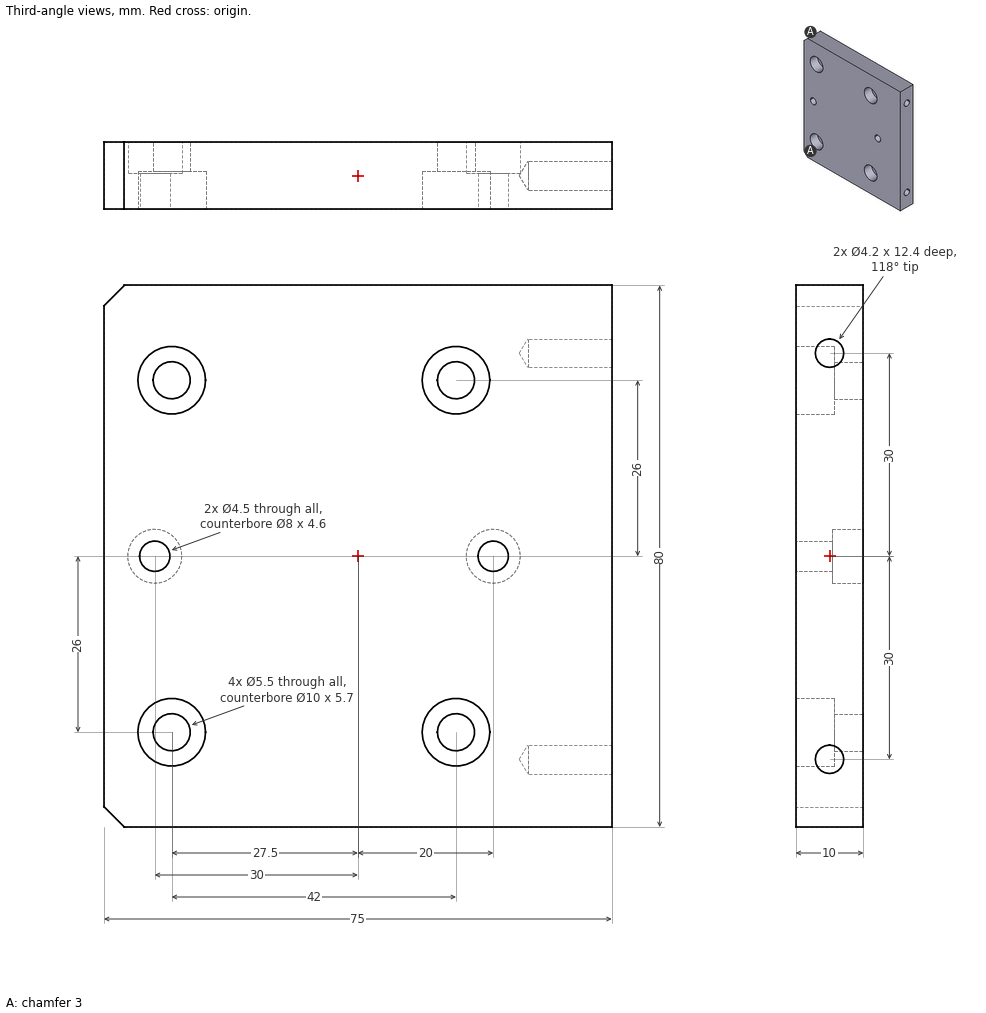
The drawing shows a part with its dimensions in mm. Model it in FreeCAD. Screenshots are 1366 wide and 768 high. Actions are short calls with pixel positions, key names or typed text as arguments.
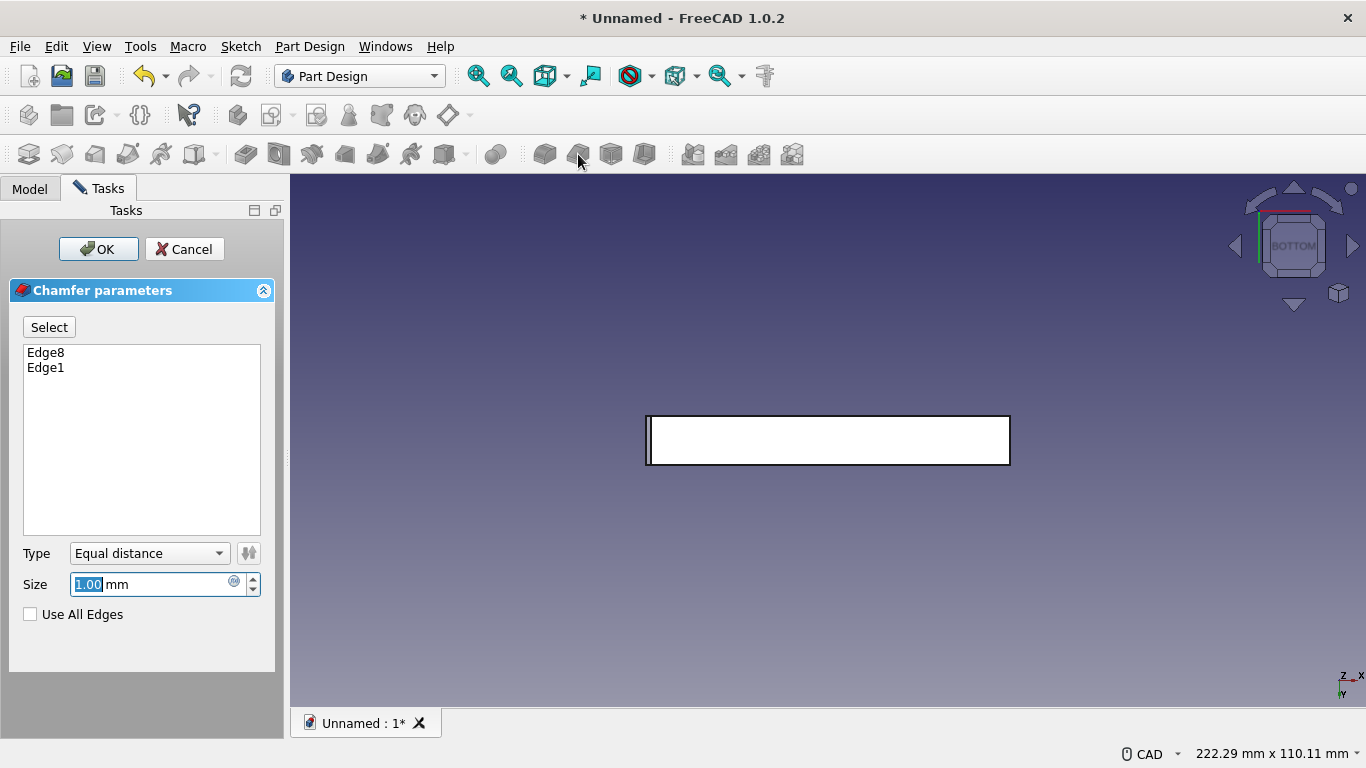
text(3)
key(Tab)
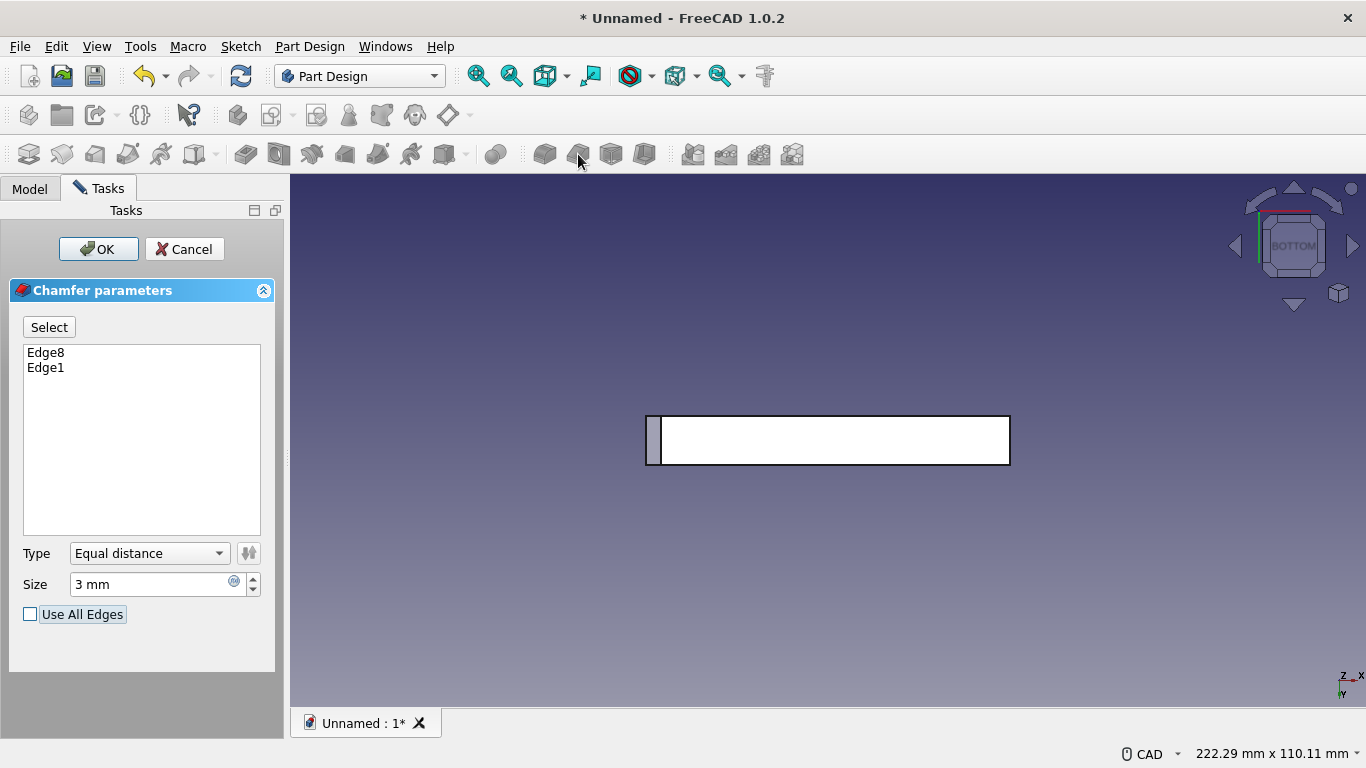
click(99, 249)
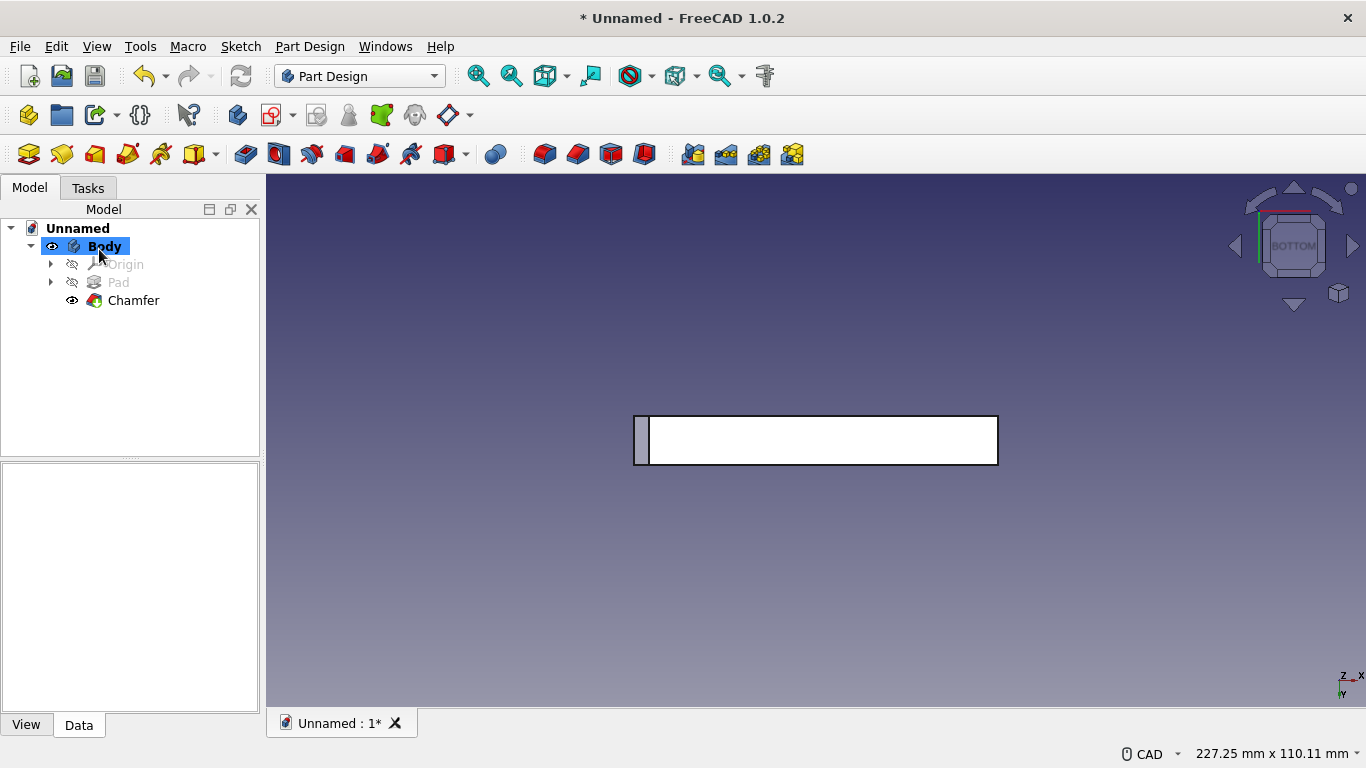
click(479, 76)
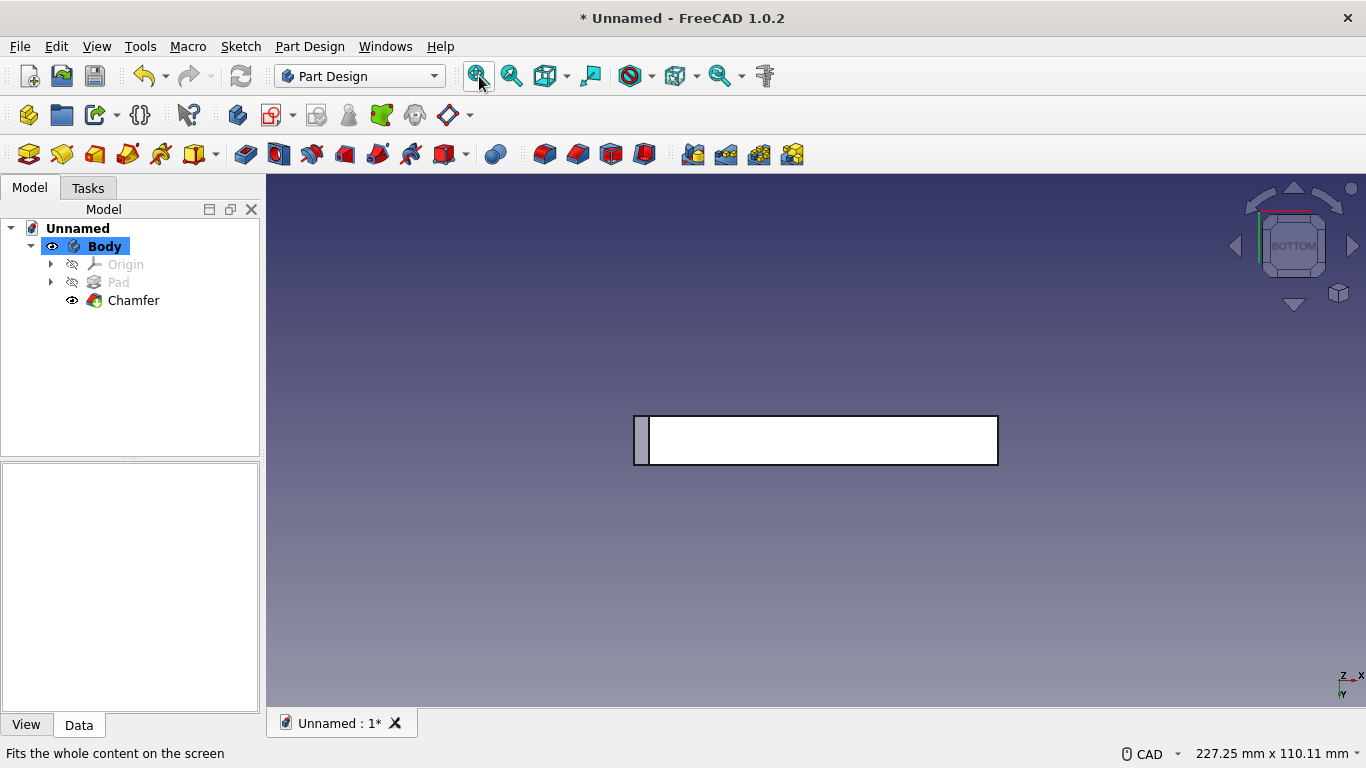
key(0)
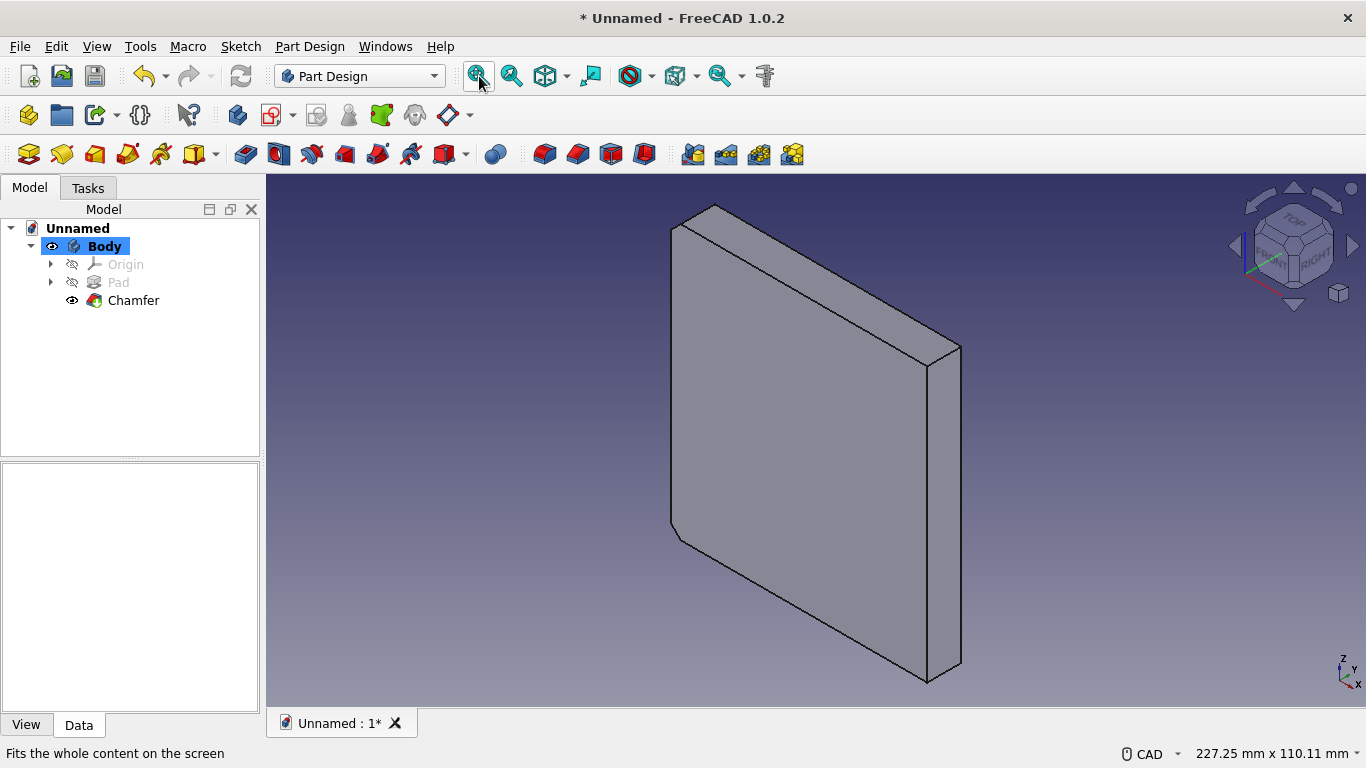
click(944, 468)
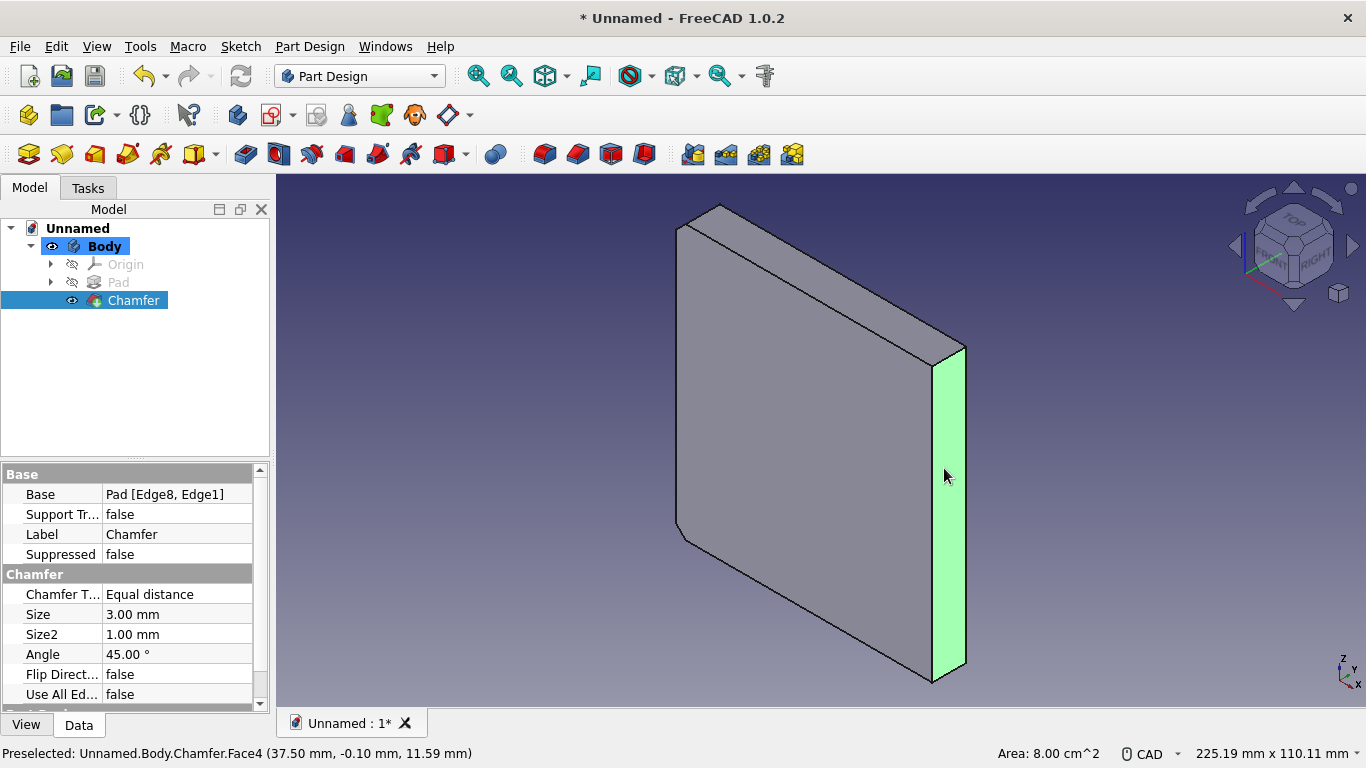
click(270, 116)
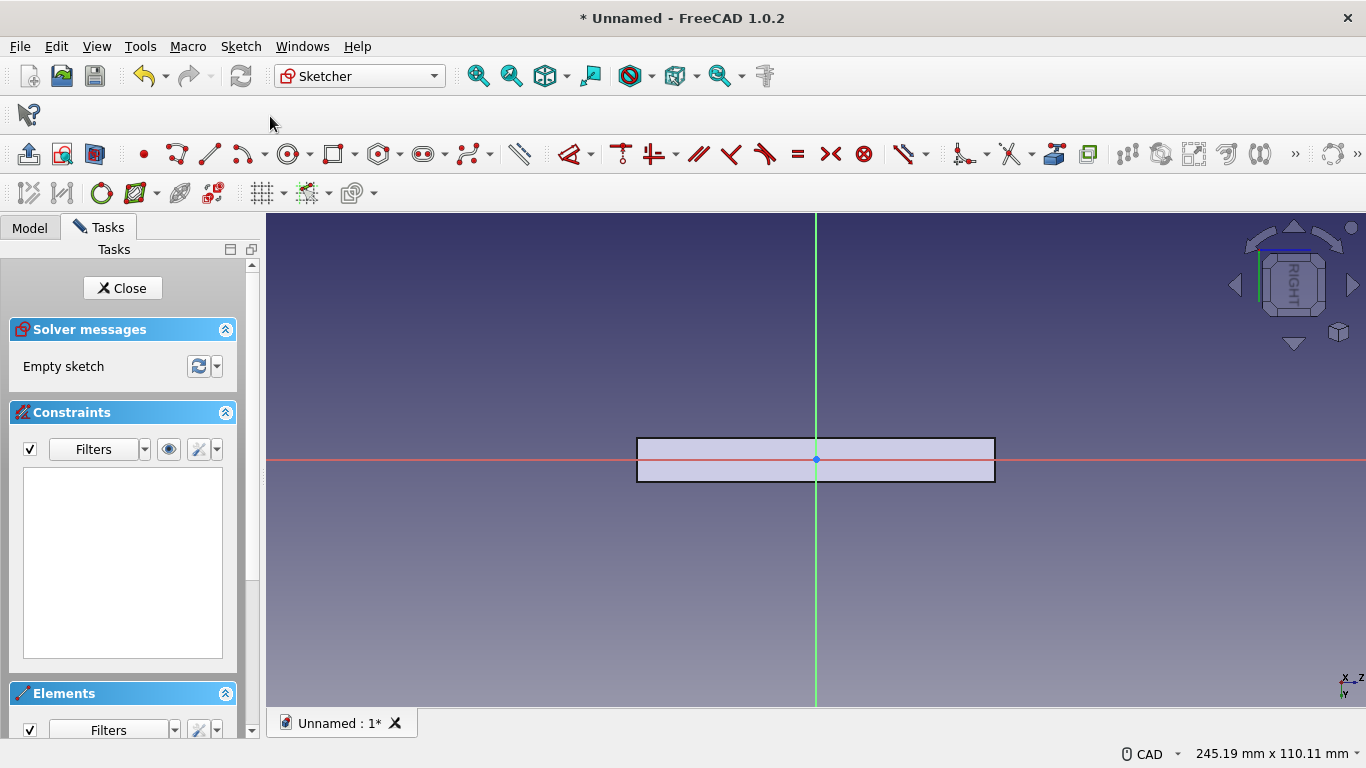
scroll(872, 460, up, 4)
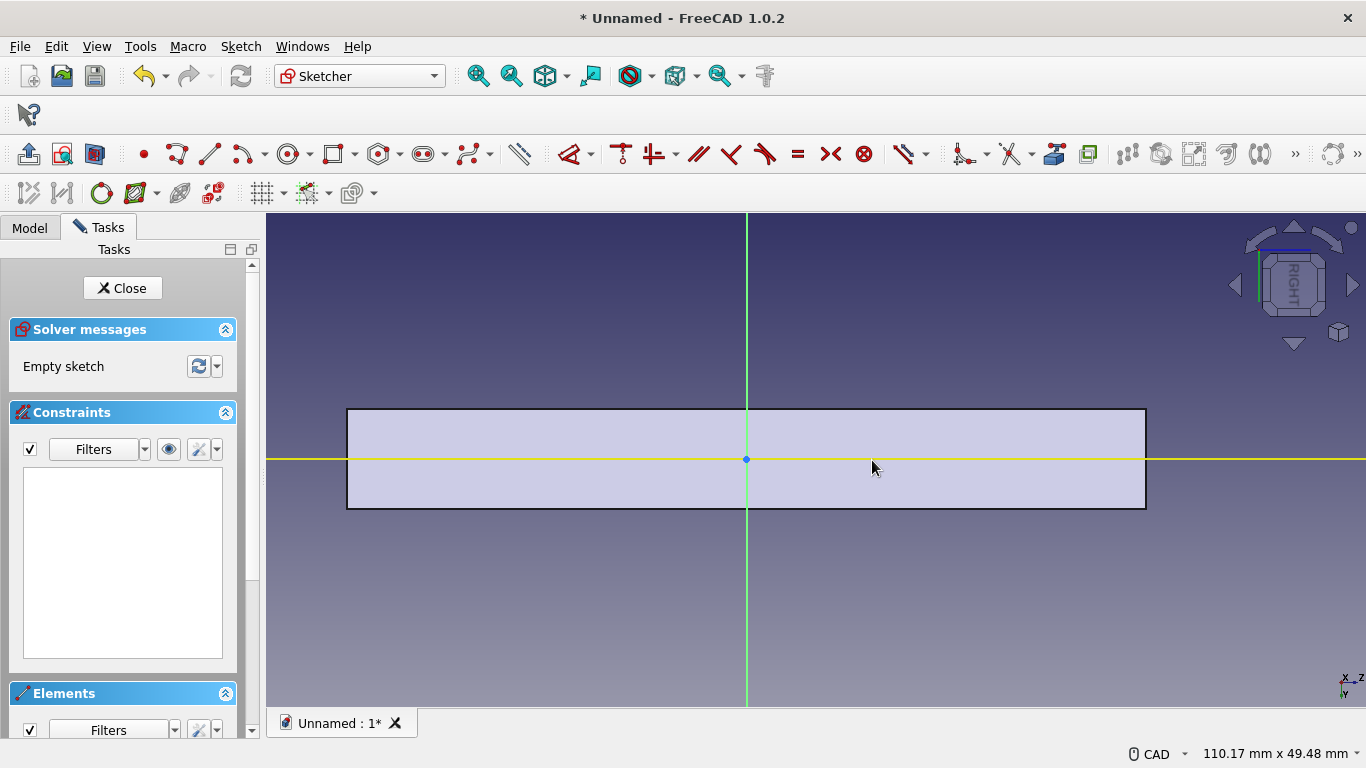
click(288, 154)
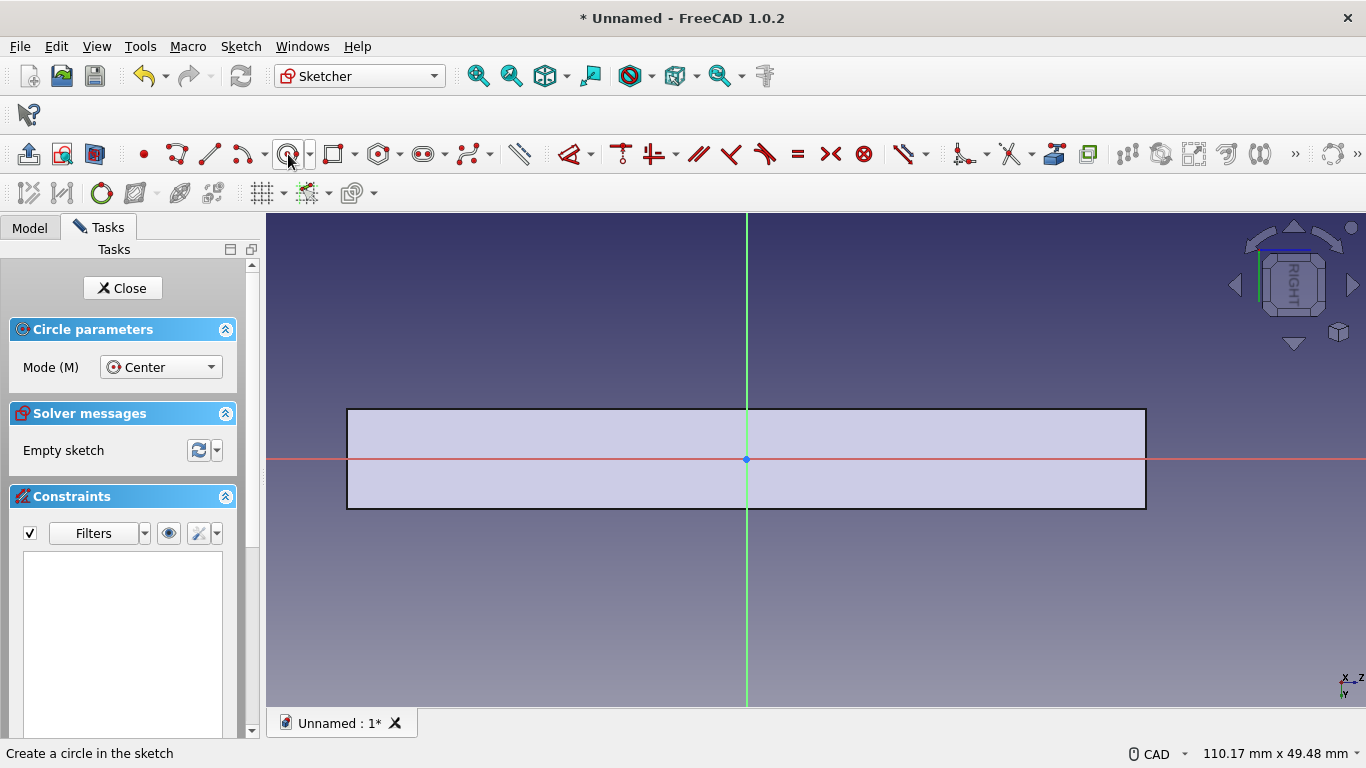
click(1046, 459)
click(1061, 445)